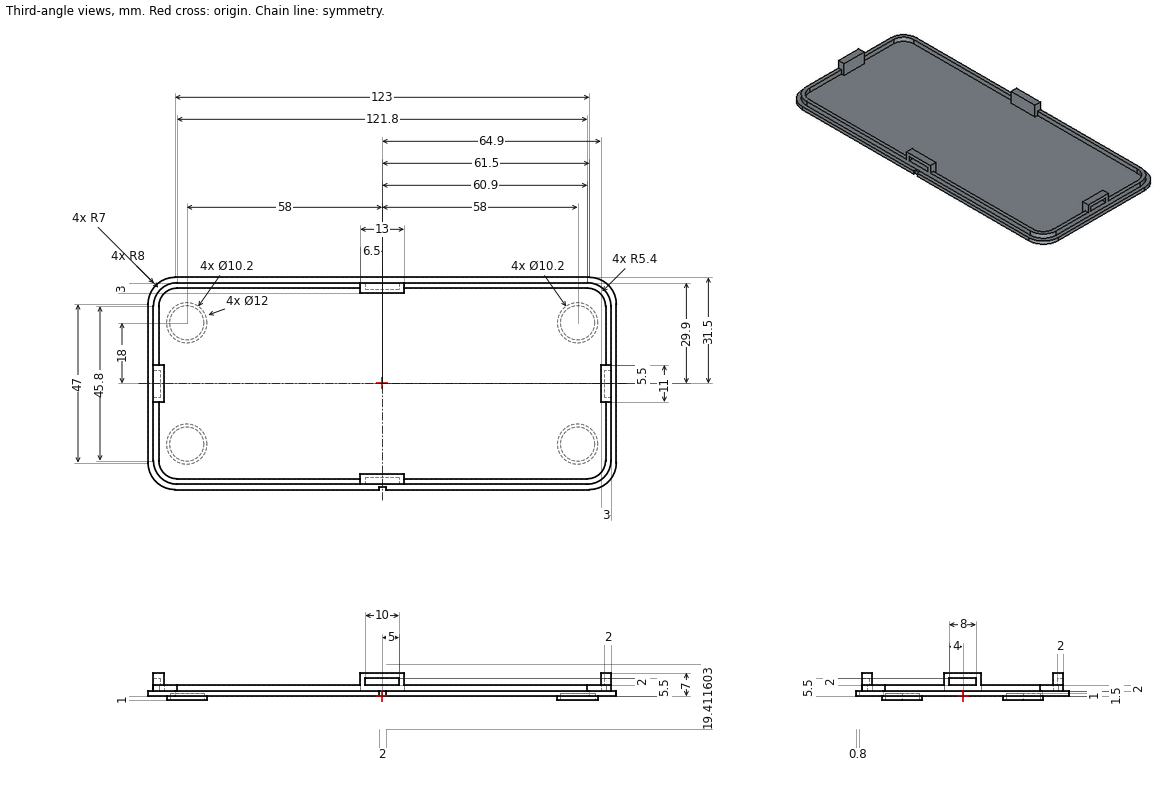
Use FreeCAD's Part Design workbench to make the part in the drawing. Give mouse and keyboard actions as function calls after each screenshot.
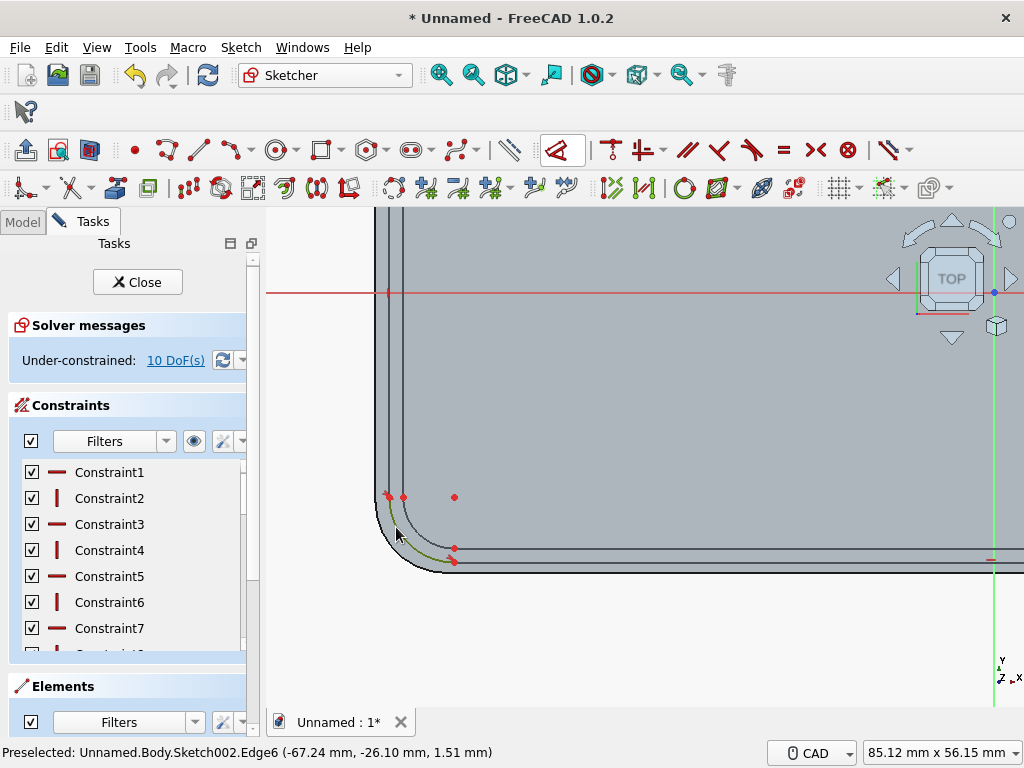
scroll(396, 528, down, 6)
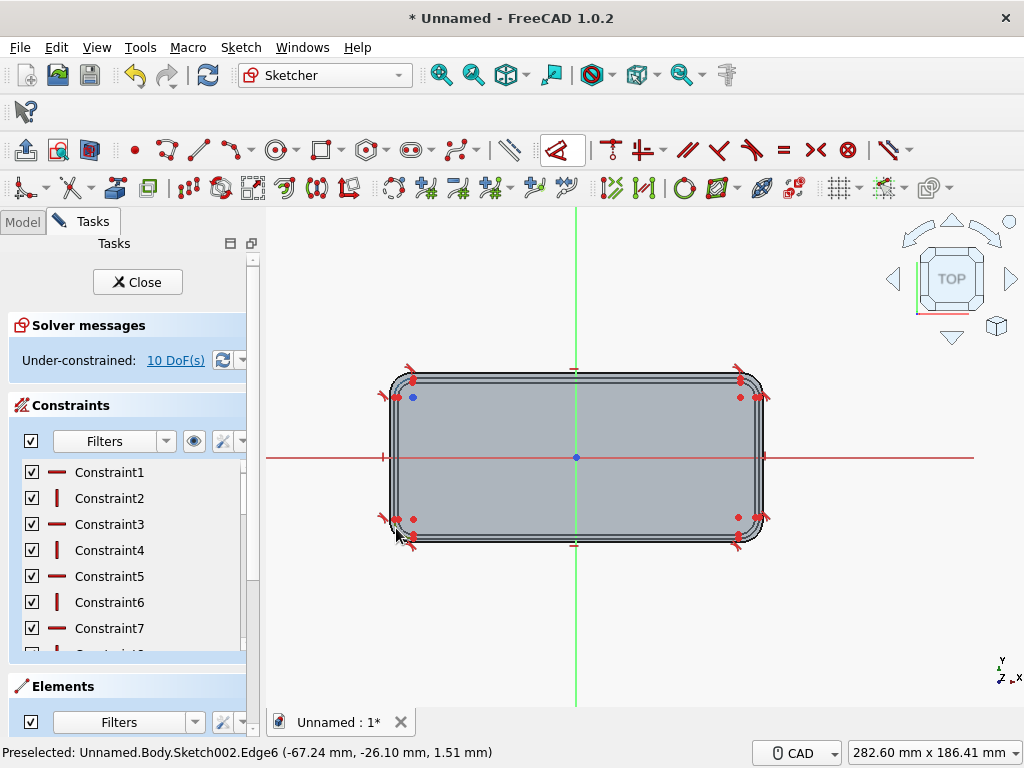
scroll(748, 537, up, 6)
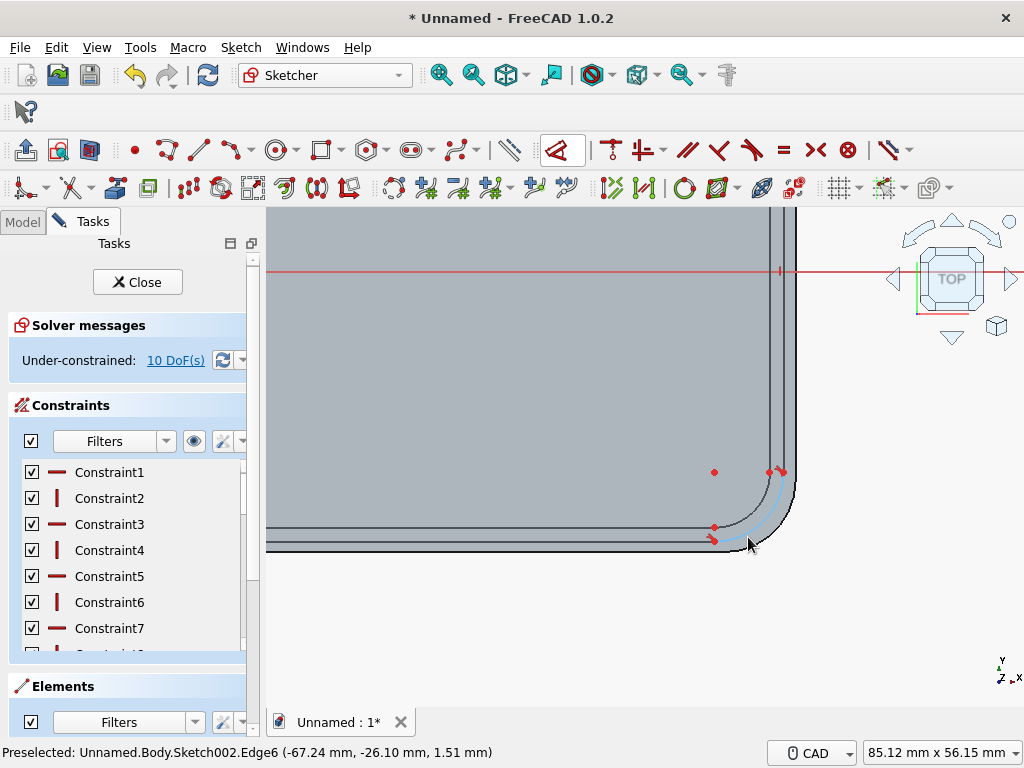
click(746, 534)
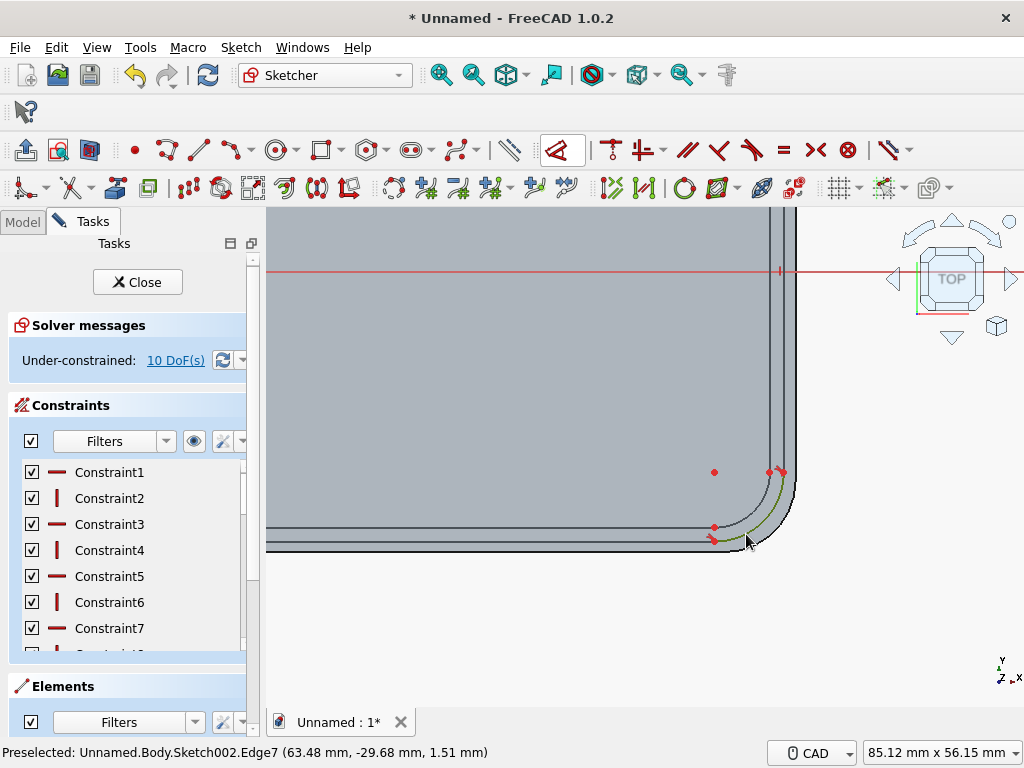
scroll(749, 537, down, 6)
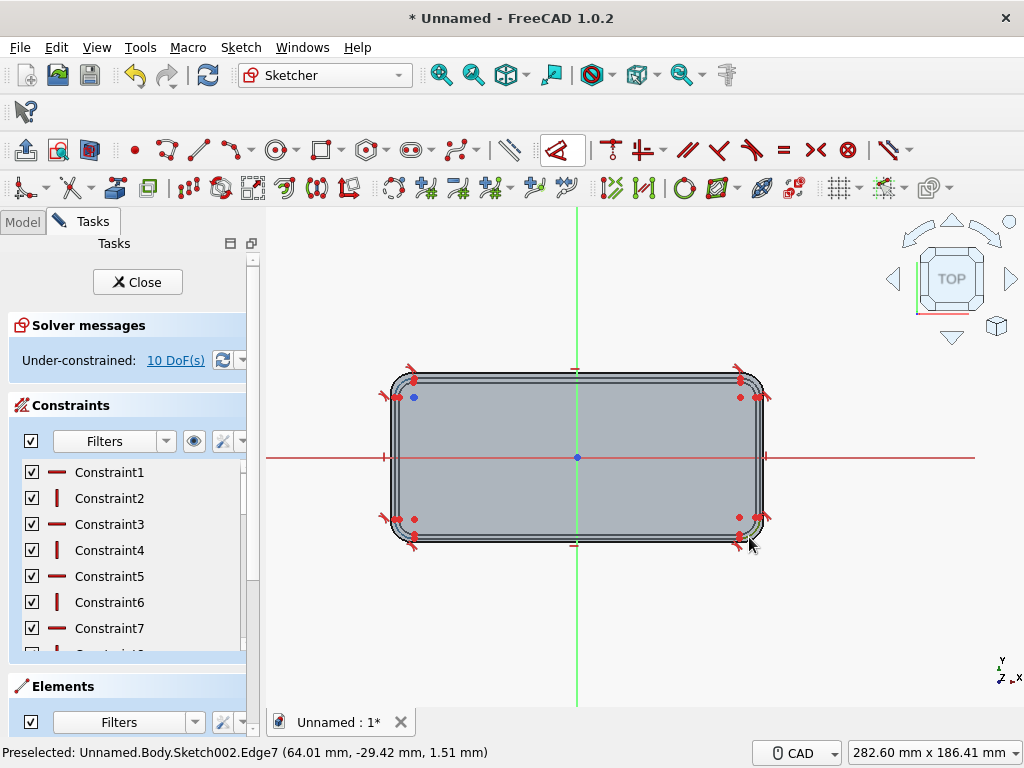
scroll(758, 389, up, 6)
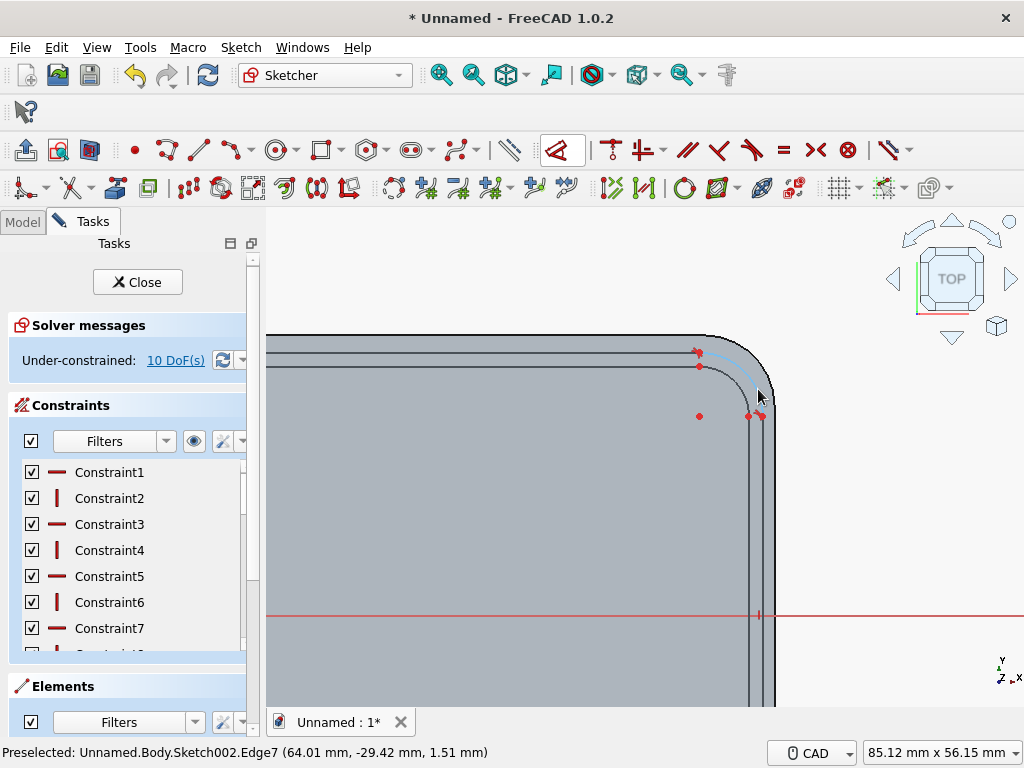
click(756, 387)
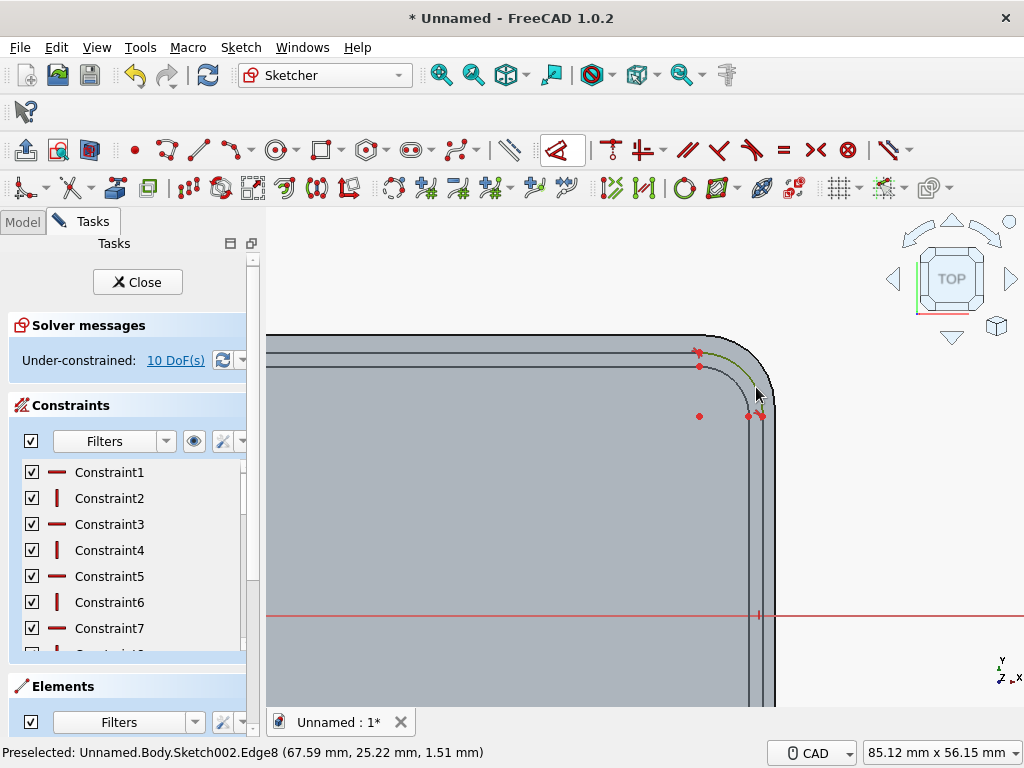
click(784, 150)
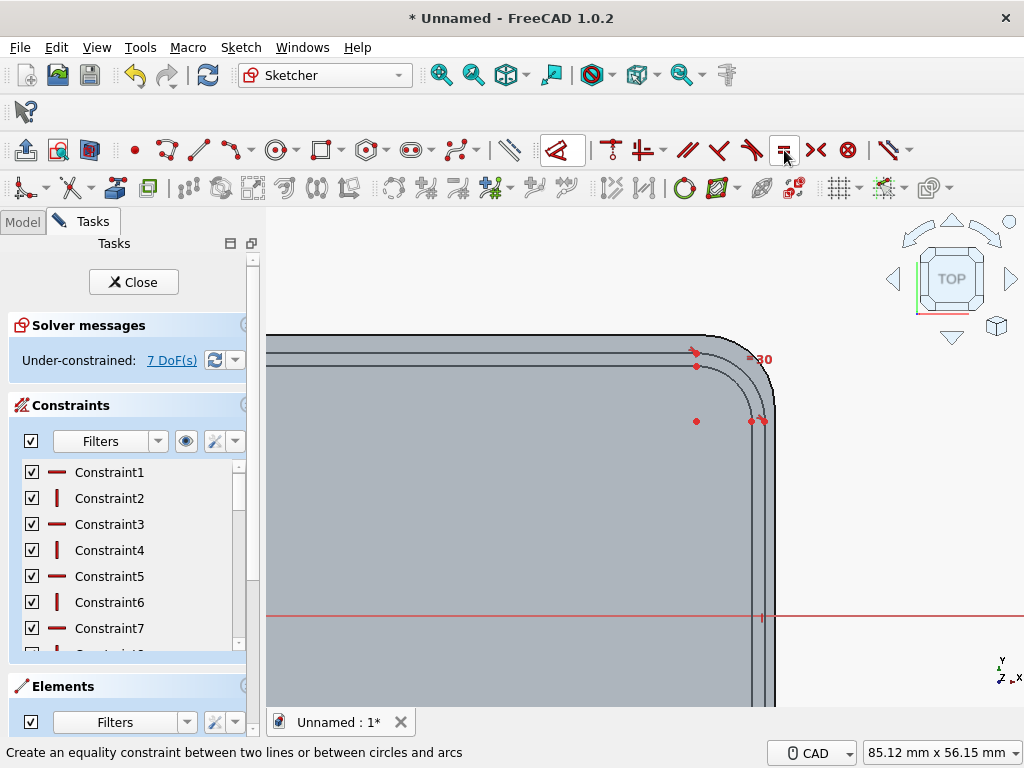
click(746, 397)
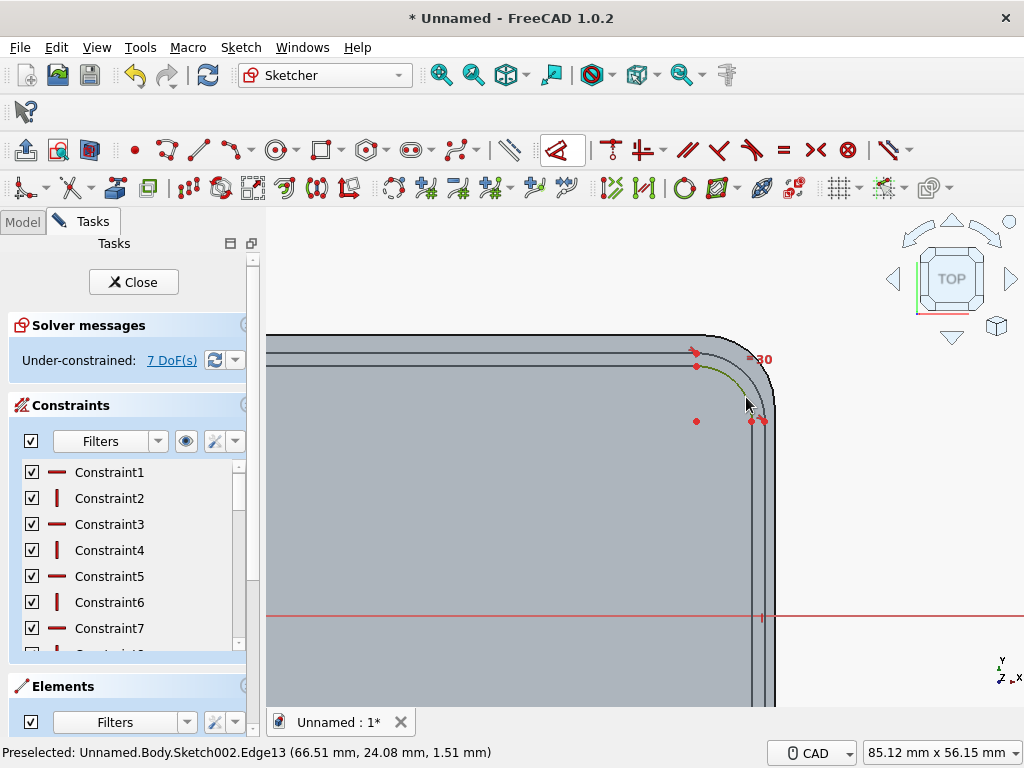
scroll(758, 389, down, 6)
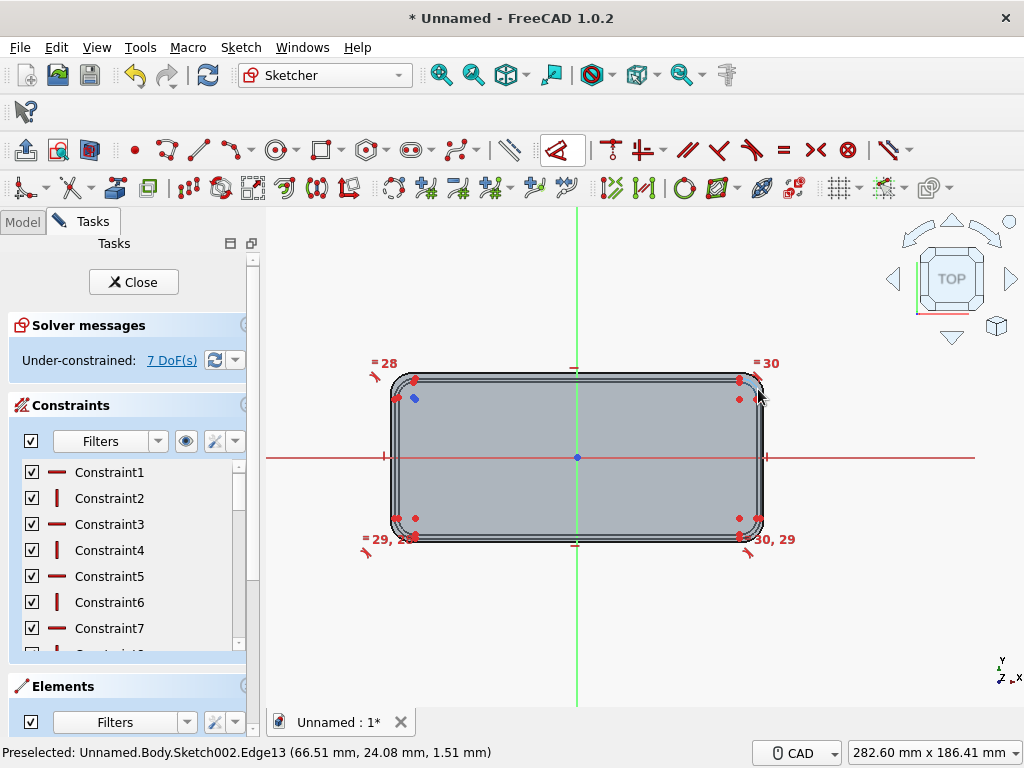
scroll(407, 384, up, 8)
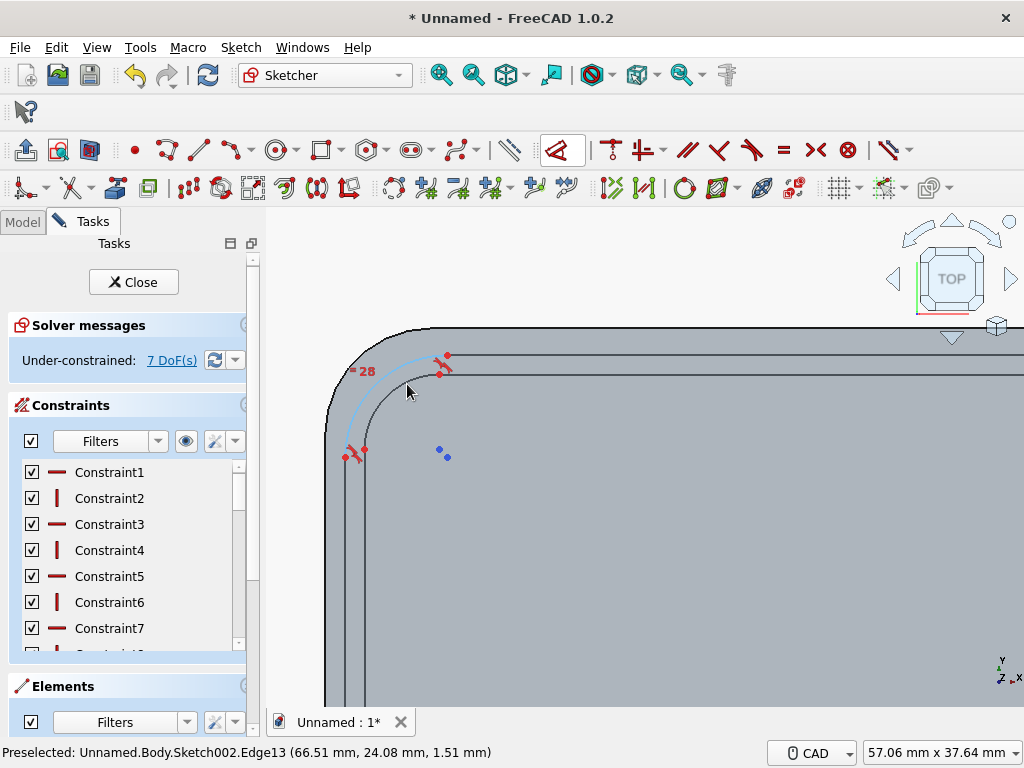
click(405, 383)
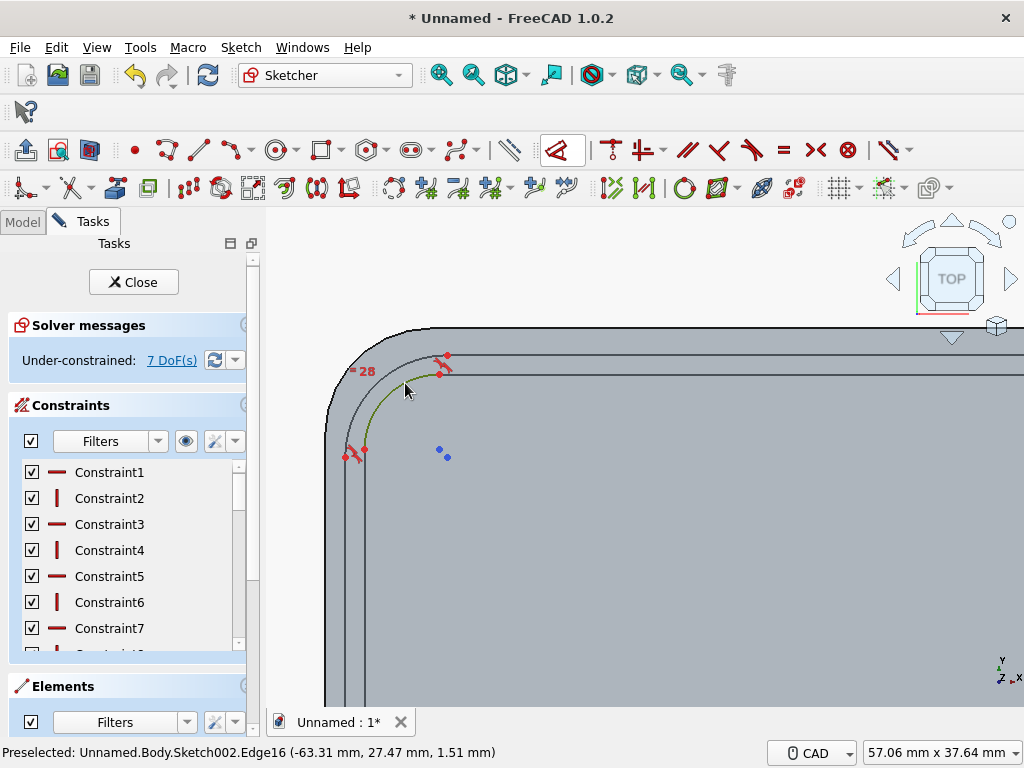
key(e)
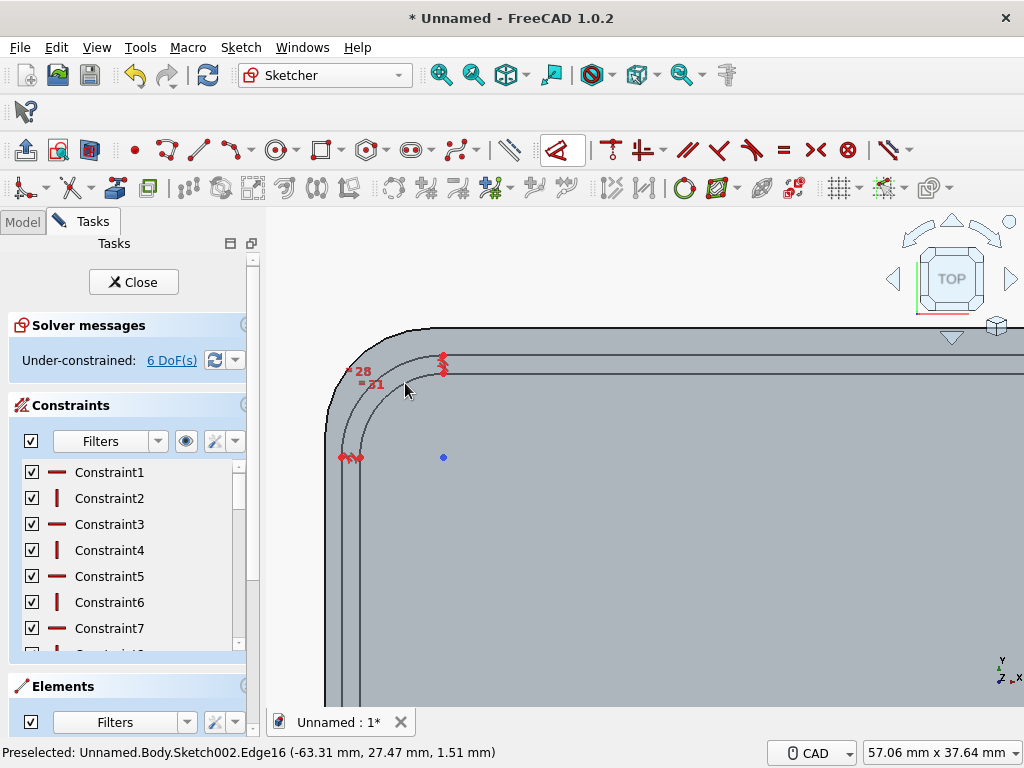
click(397, 366)